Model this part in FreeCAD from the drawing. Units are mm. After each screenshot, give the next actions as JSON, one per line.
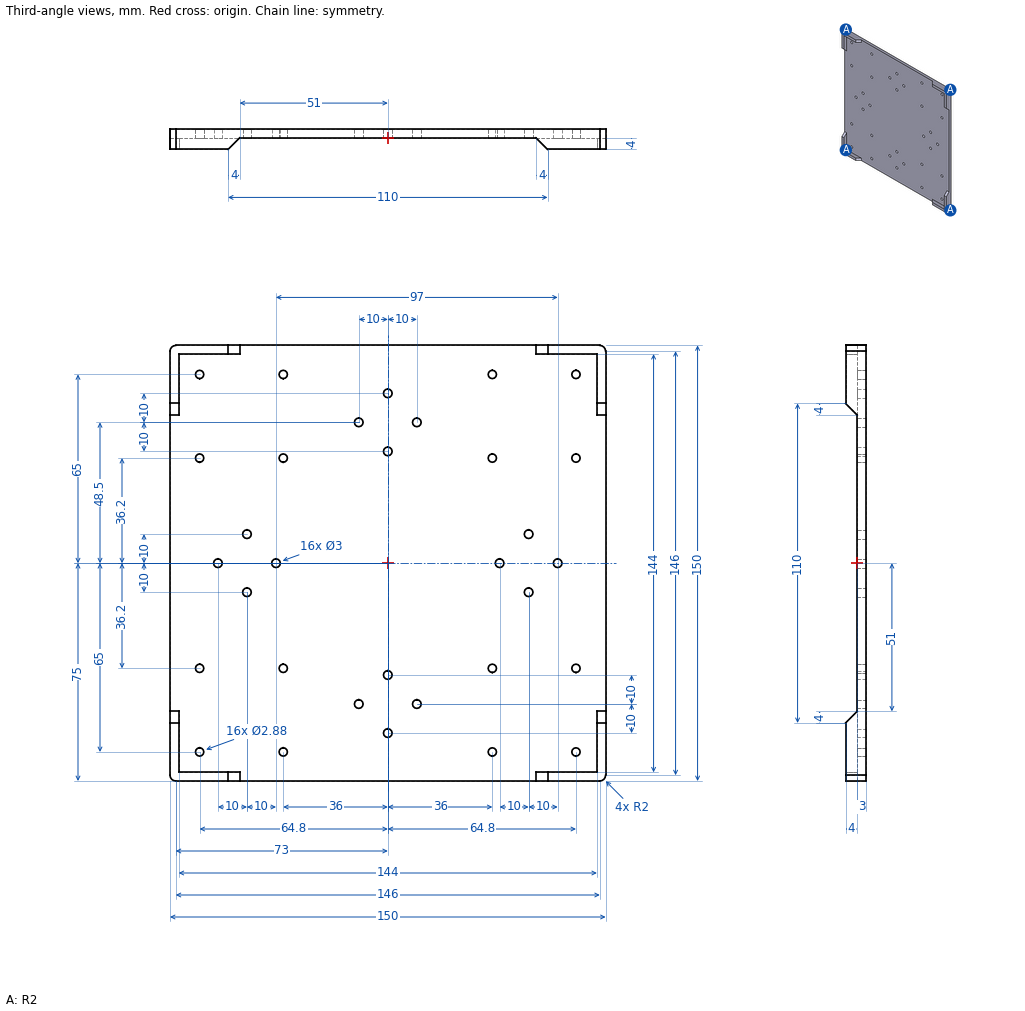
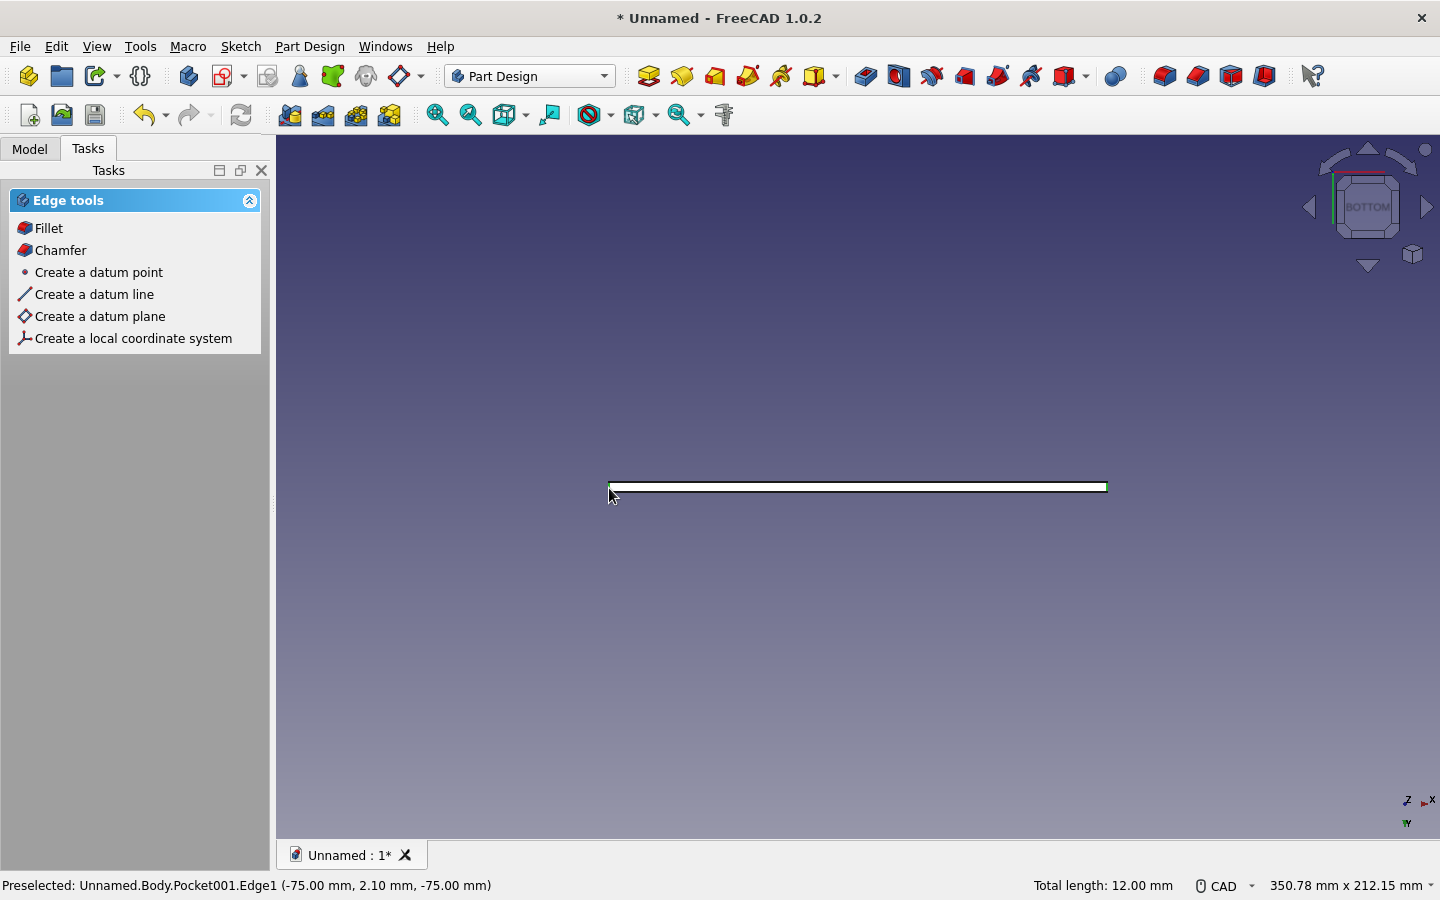
{"action": "left_click", "coordinate": [1165, 76]}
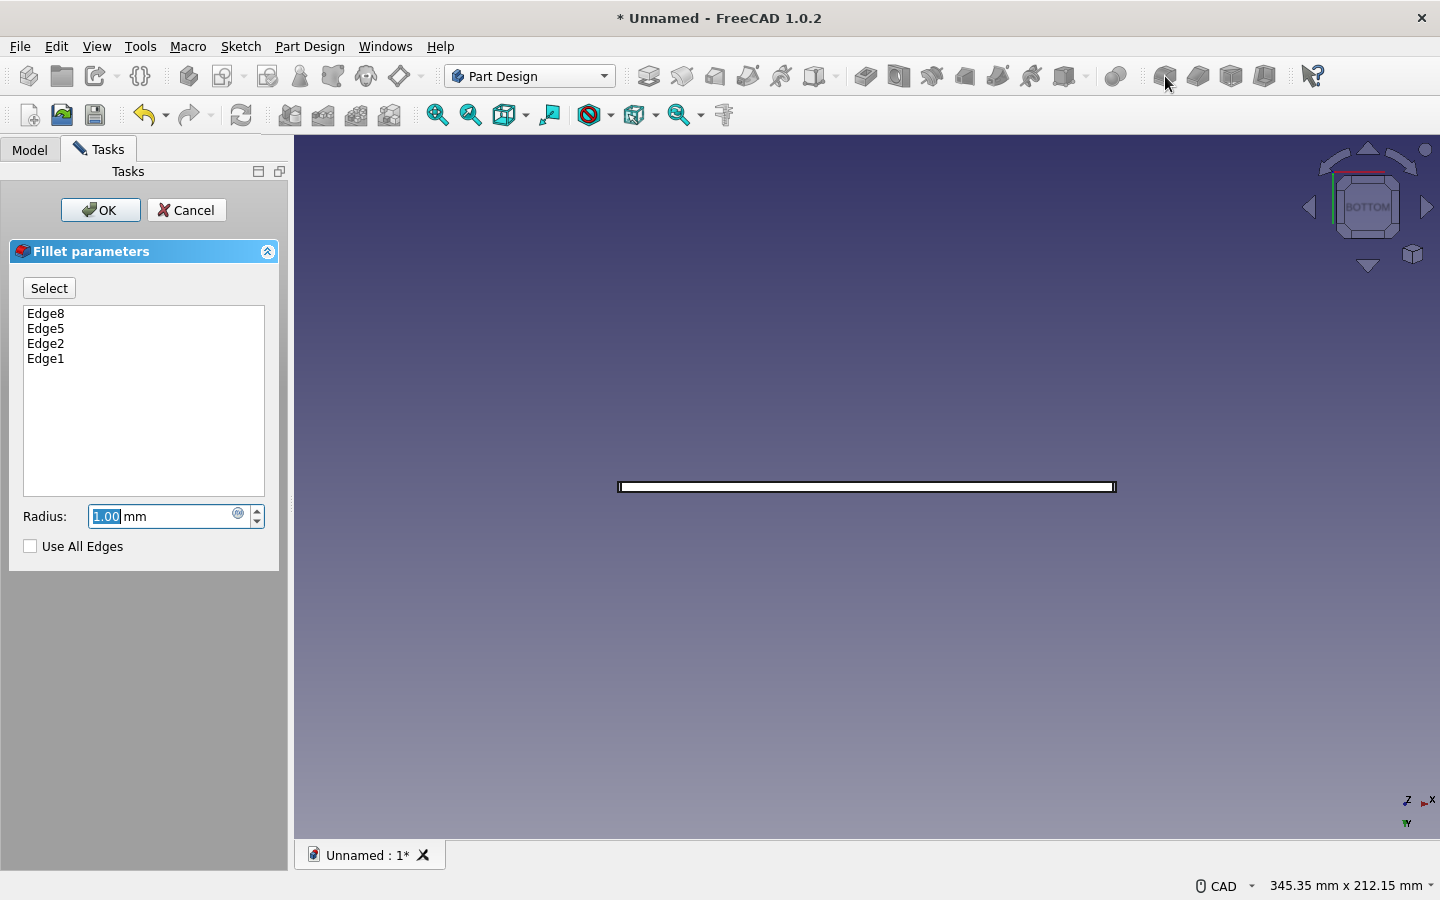
{"action": "type", "text": "2"}
{"action": "key", "text": "Tab"}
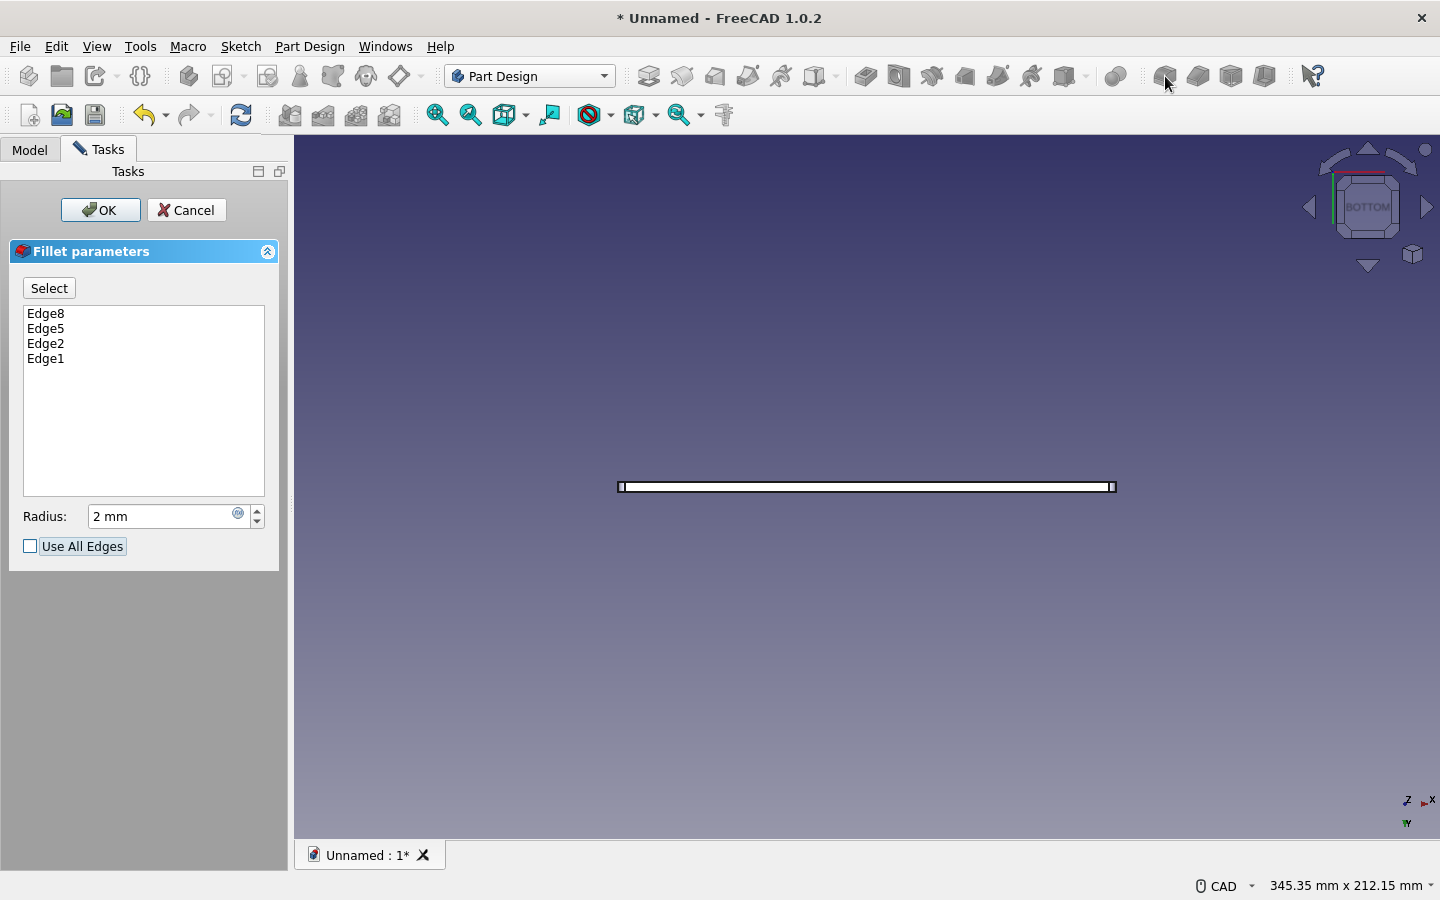
{"action": "left_click", "coordinate": [101, 210]}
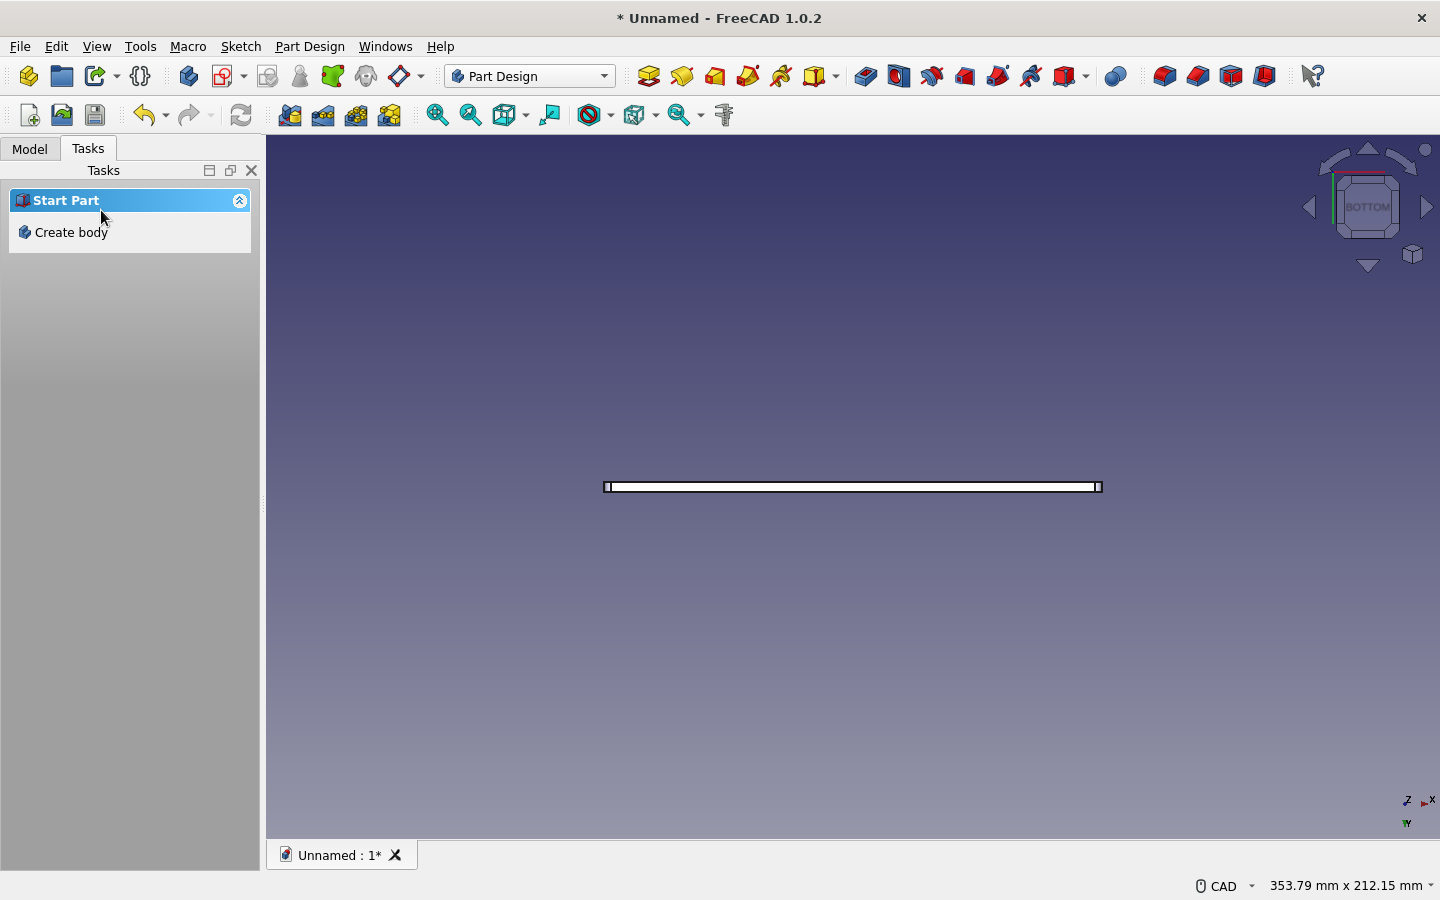
{"action": "key", "text": "v f"}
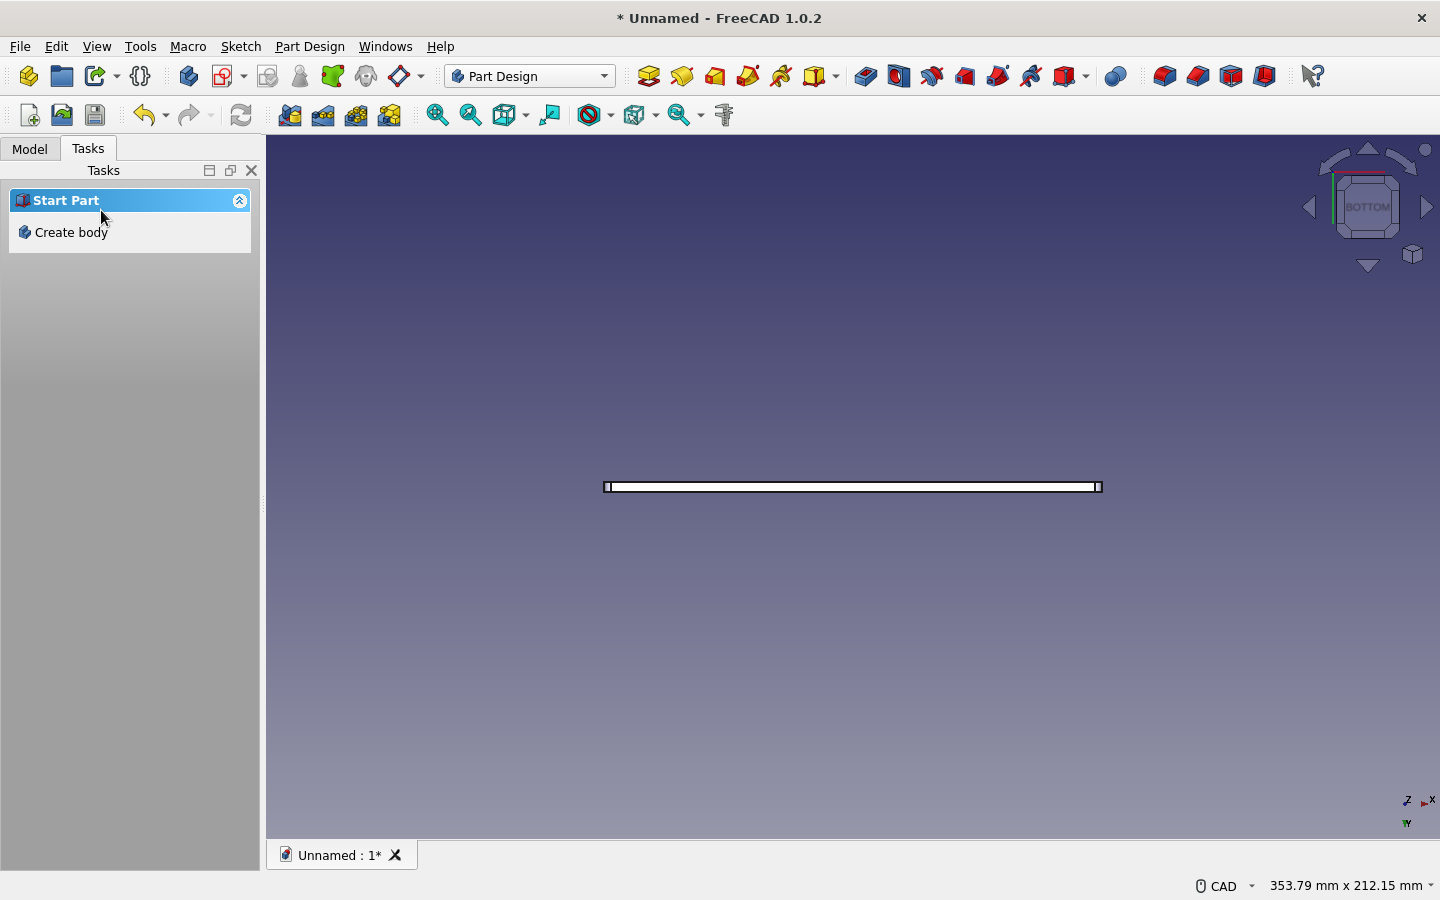
{"action": "key", "text": "0"}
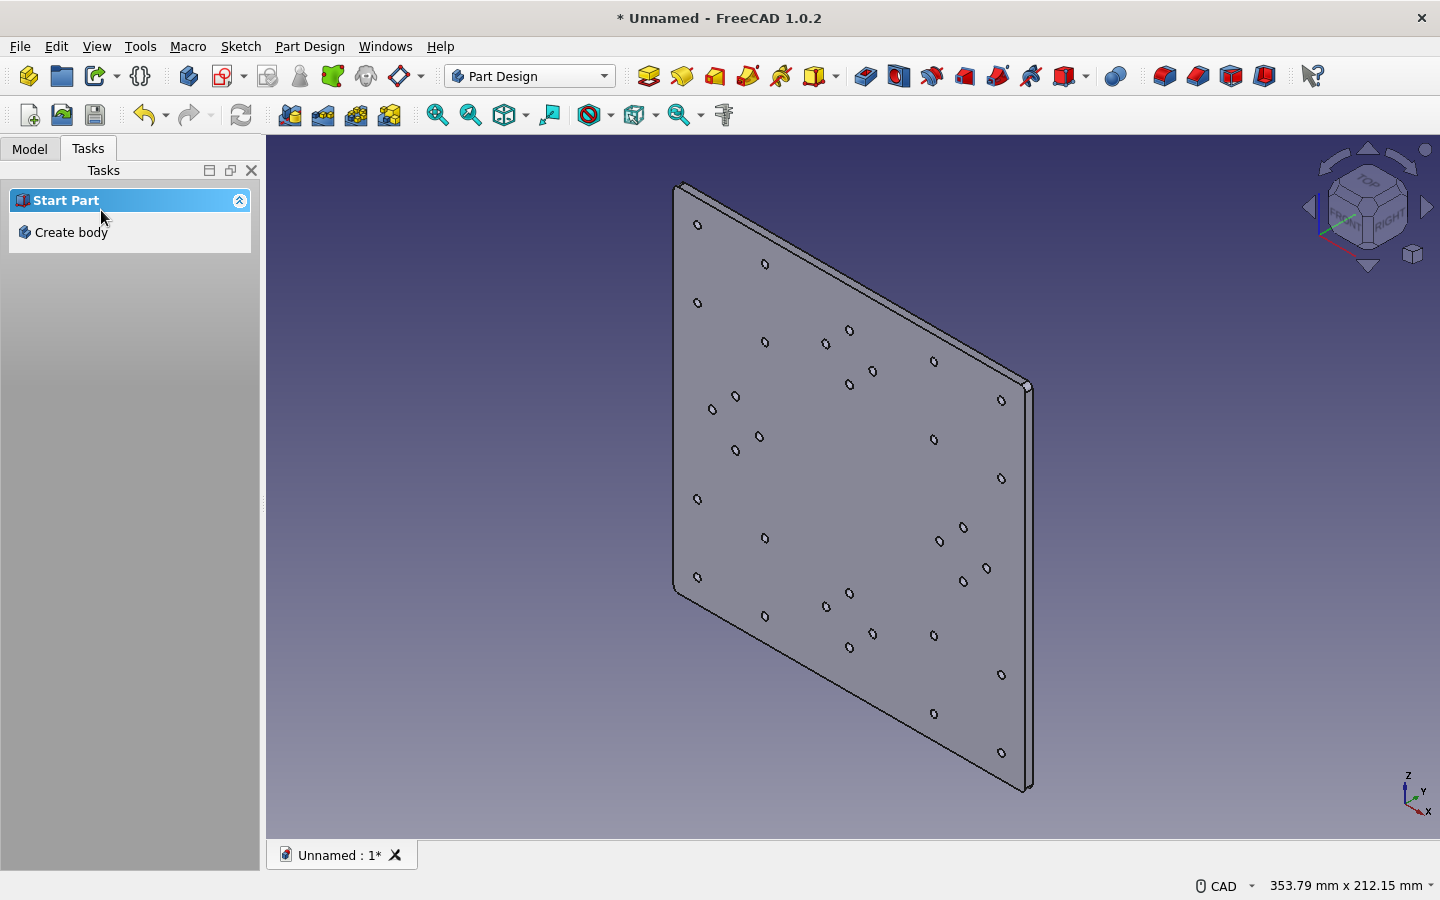
{"action": "left_click", "coordinate": [849, 488]}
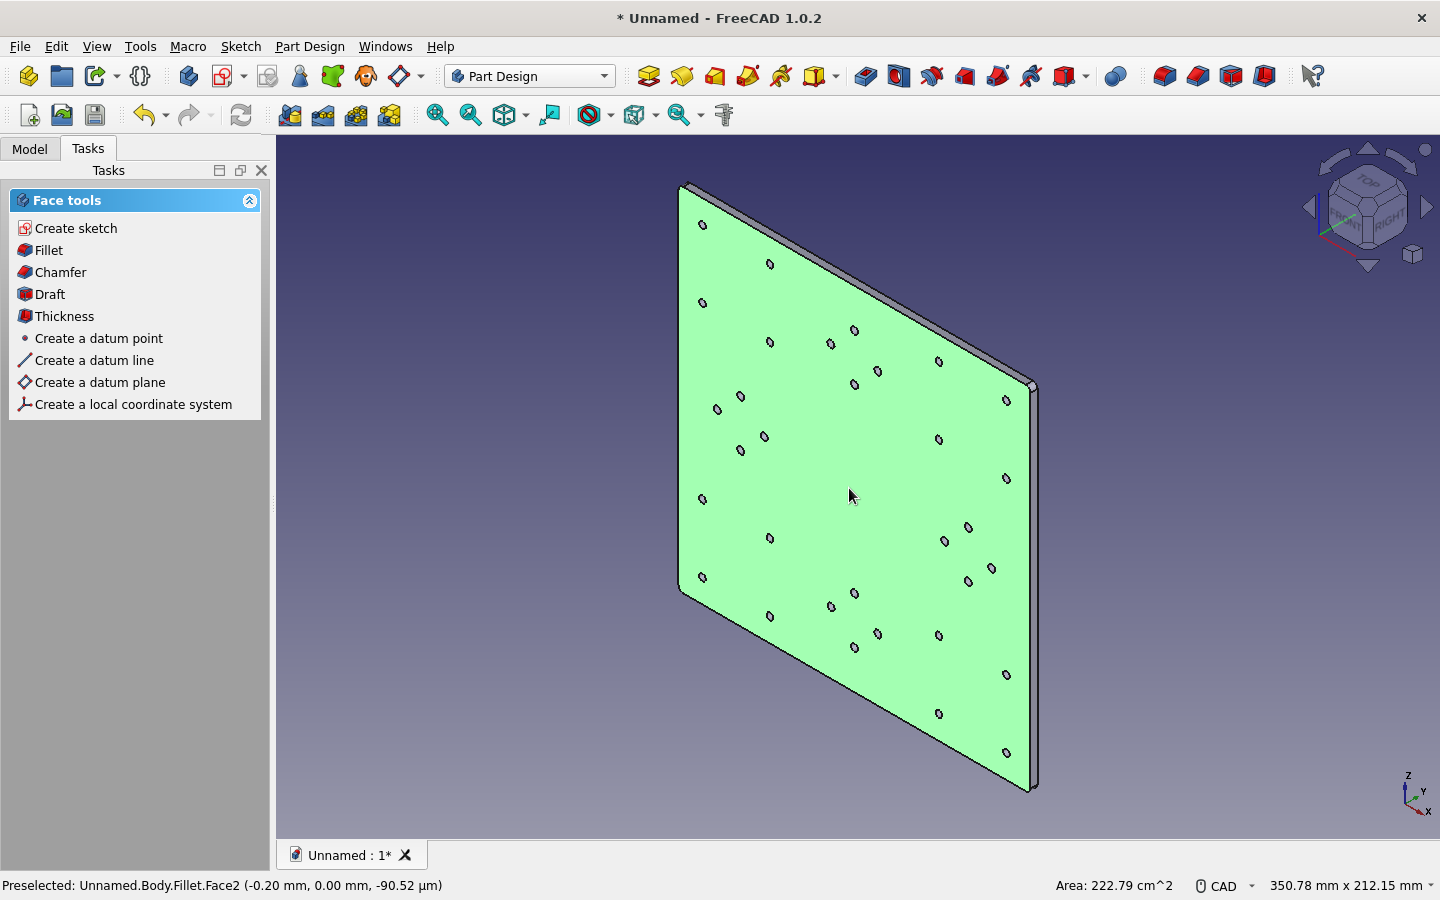
{"action": "left_click", "coordinate": [222, 76]}